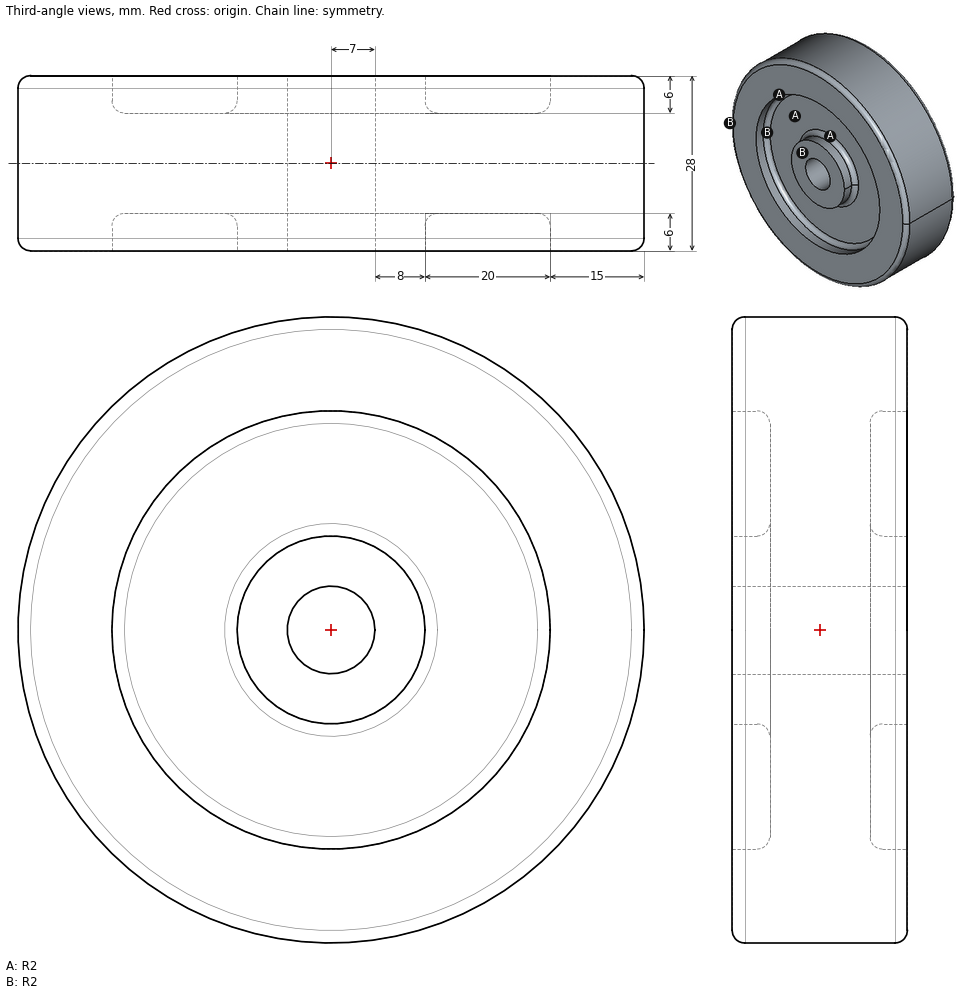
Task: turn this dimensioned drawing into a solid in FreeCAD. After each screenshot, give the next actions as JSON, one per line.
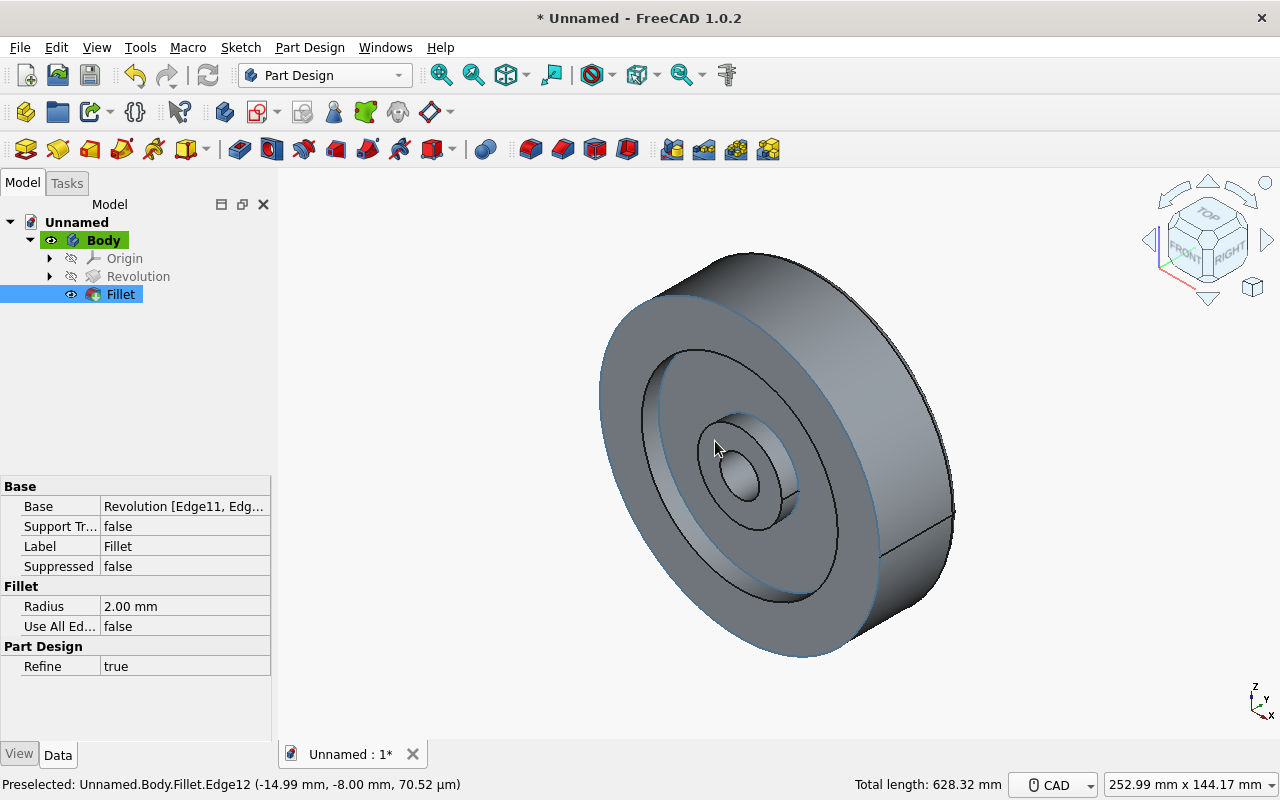
{"action": "left_click", "coordinate": [532, 150]}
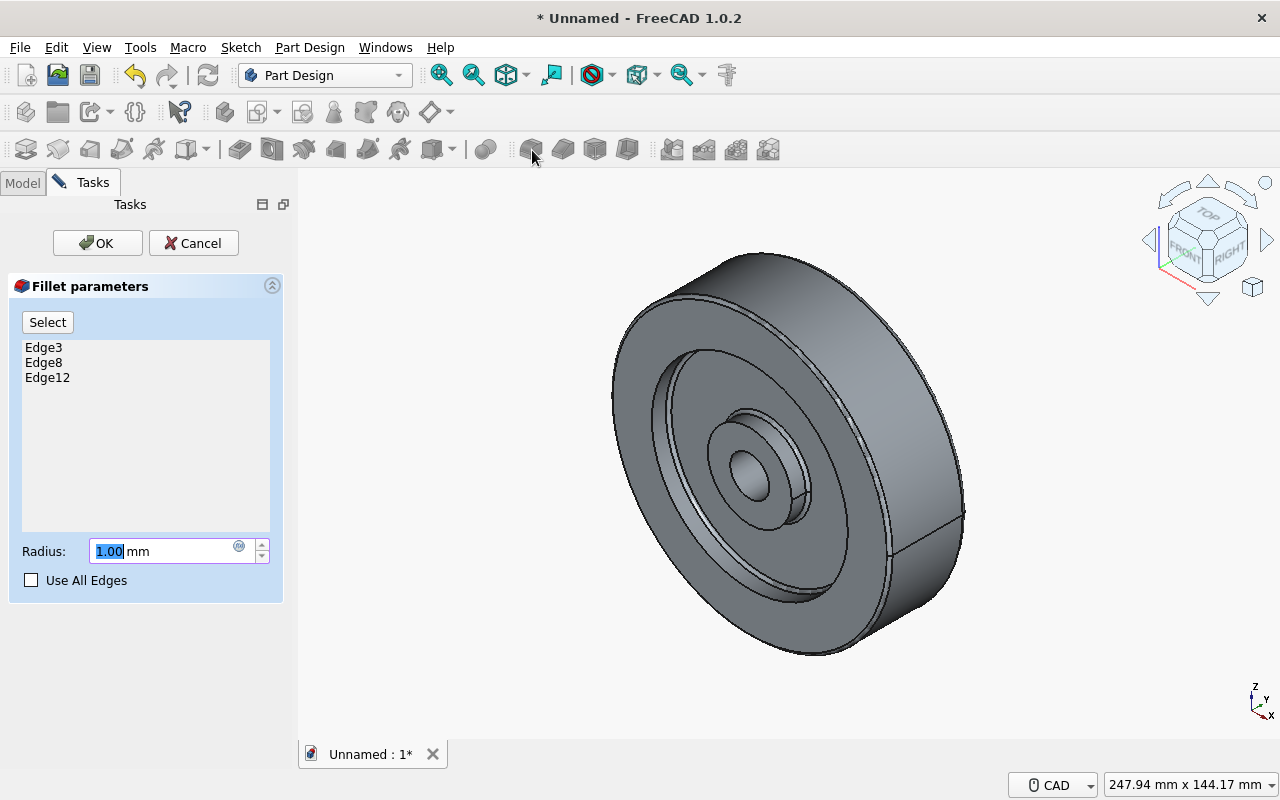
{"action": "type", "text": "2"}
{"action": "key", "text": "Tab"}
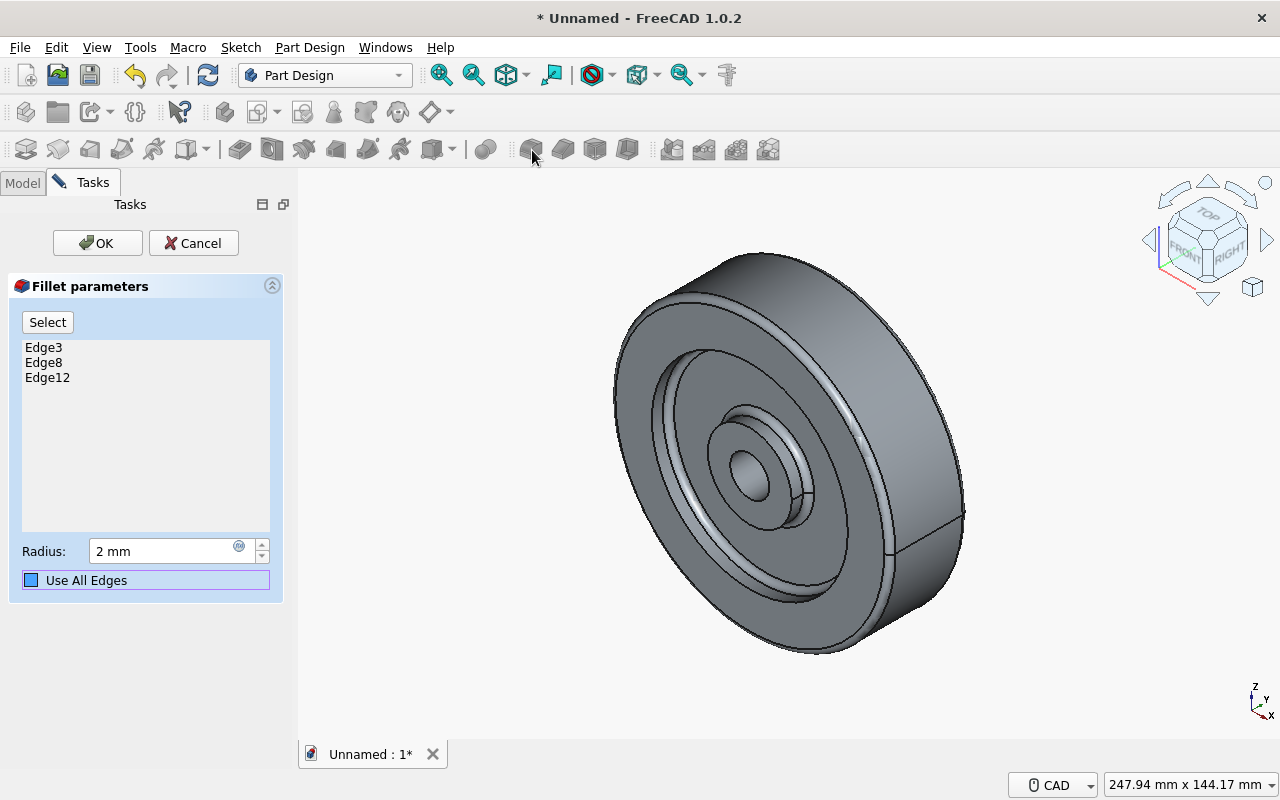
{"action": "left_click", "coordinate": [98, 243]}